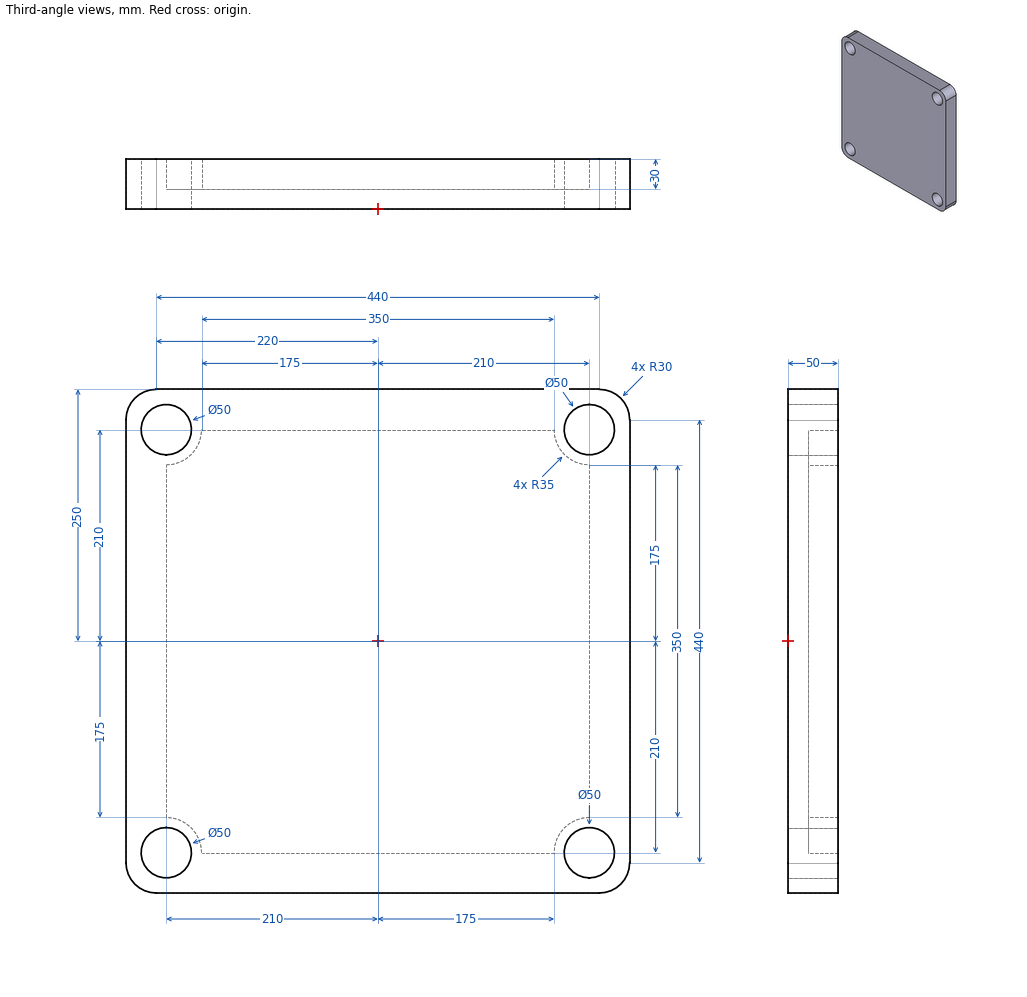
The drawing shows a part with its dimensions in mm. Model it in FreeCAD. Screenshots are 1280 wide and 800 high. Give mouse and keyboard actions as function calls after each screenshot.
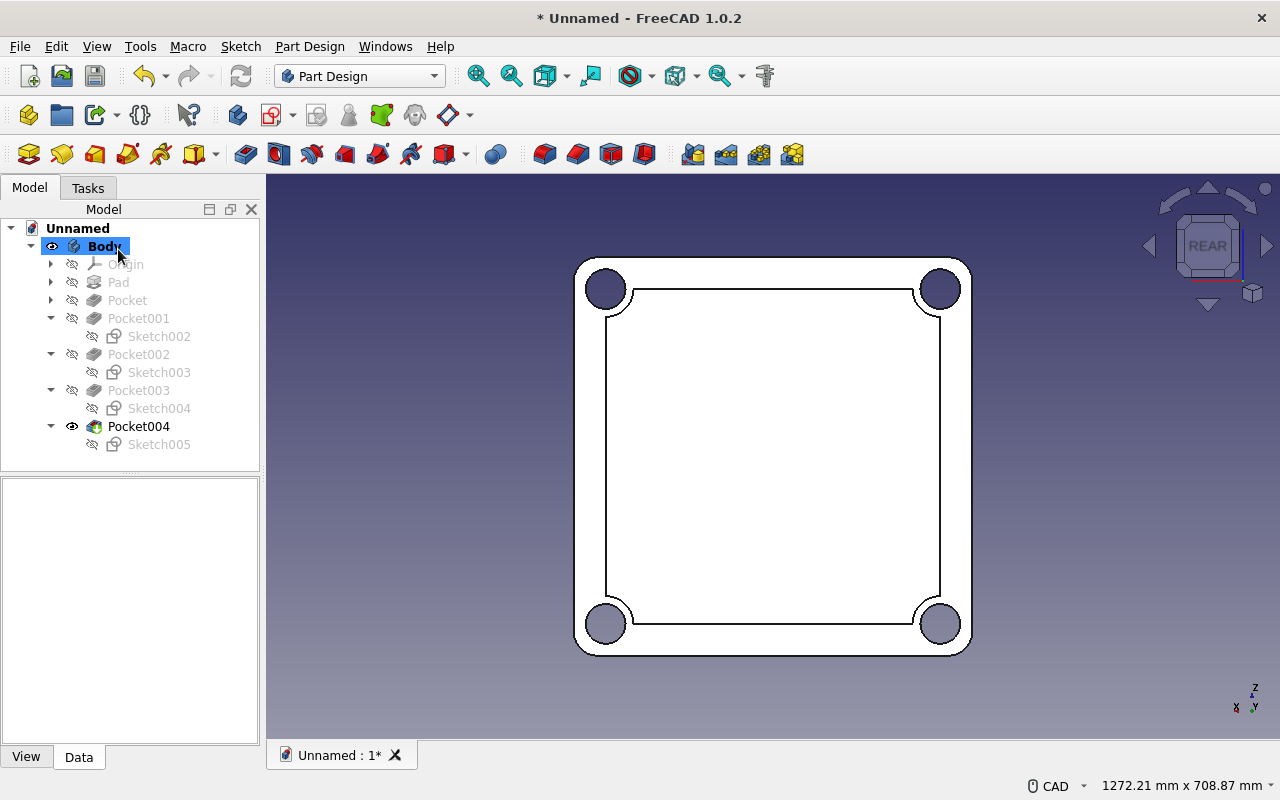
key(0)